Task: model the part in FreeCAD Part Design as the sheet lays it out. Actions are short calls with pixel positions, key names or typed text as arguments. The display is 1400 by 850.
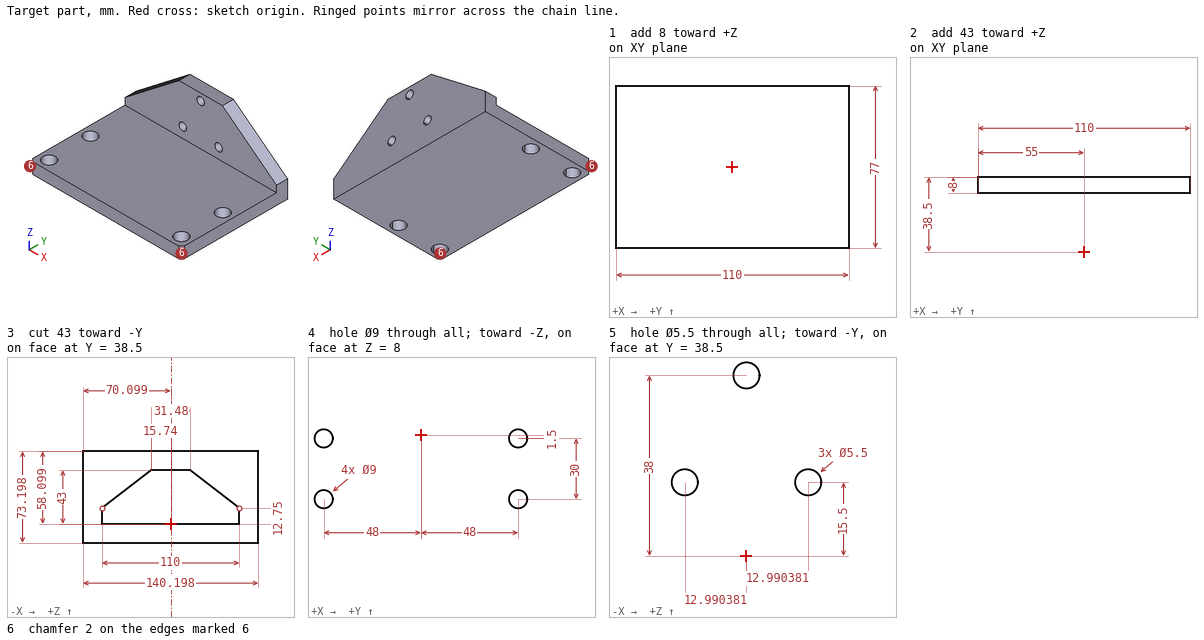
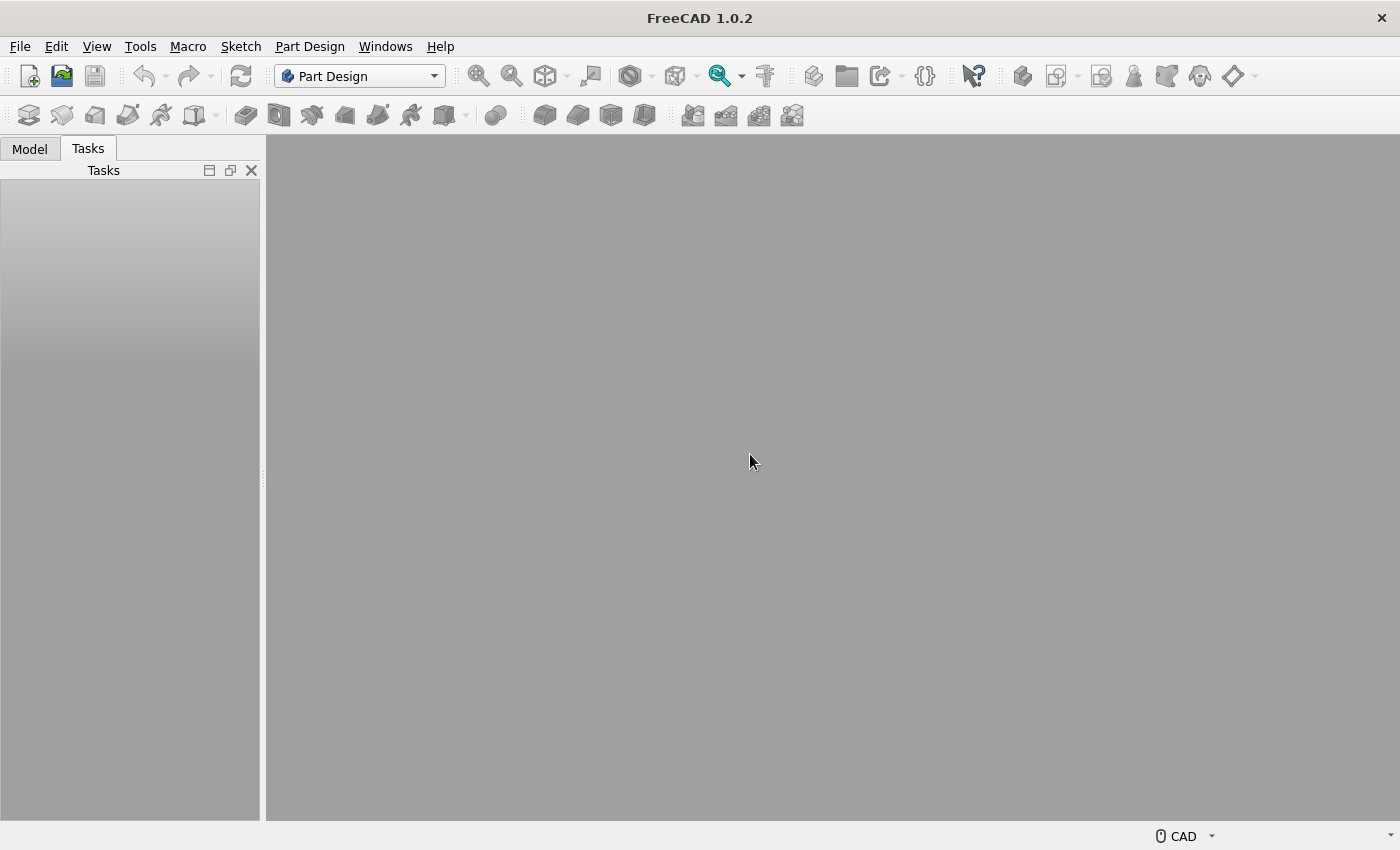
key(ctrl+n)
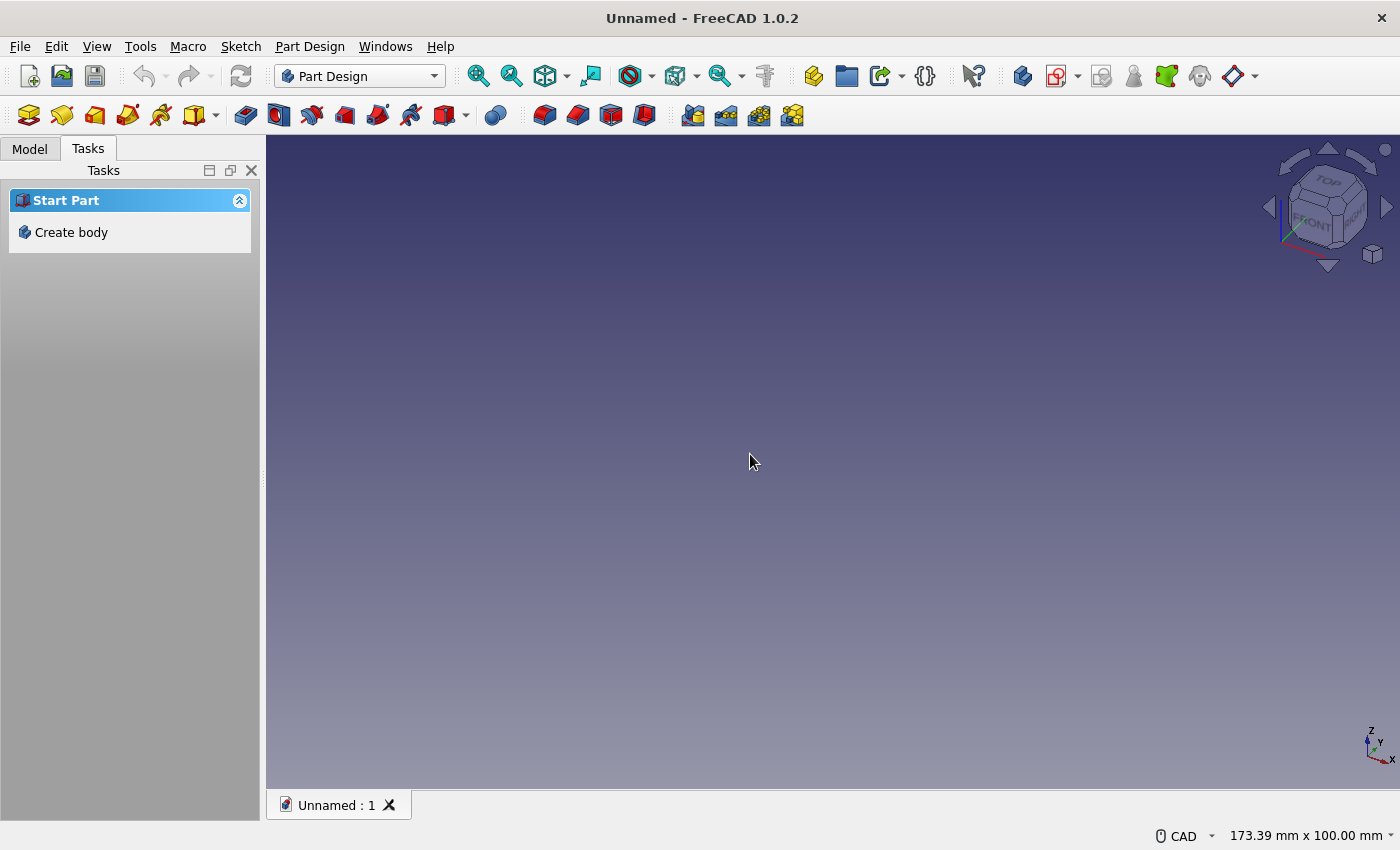
click(1056, 76)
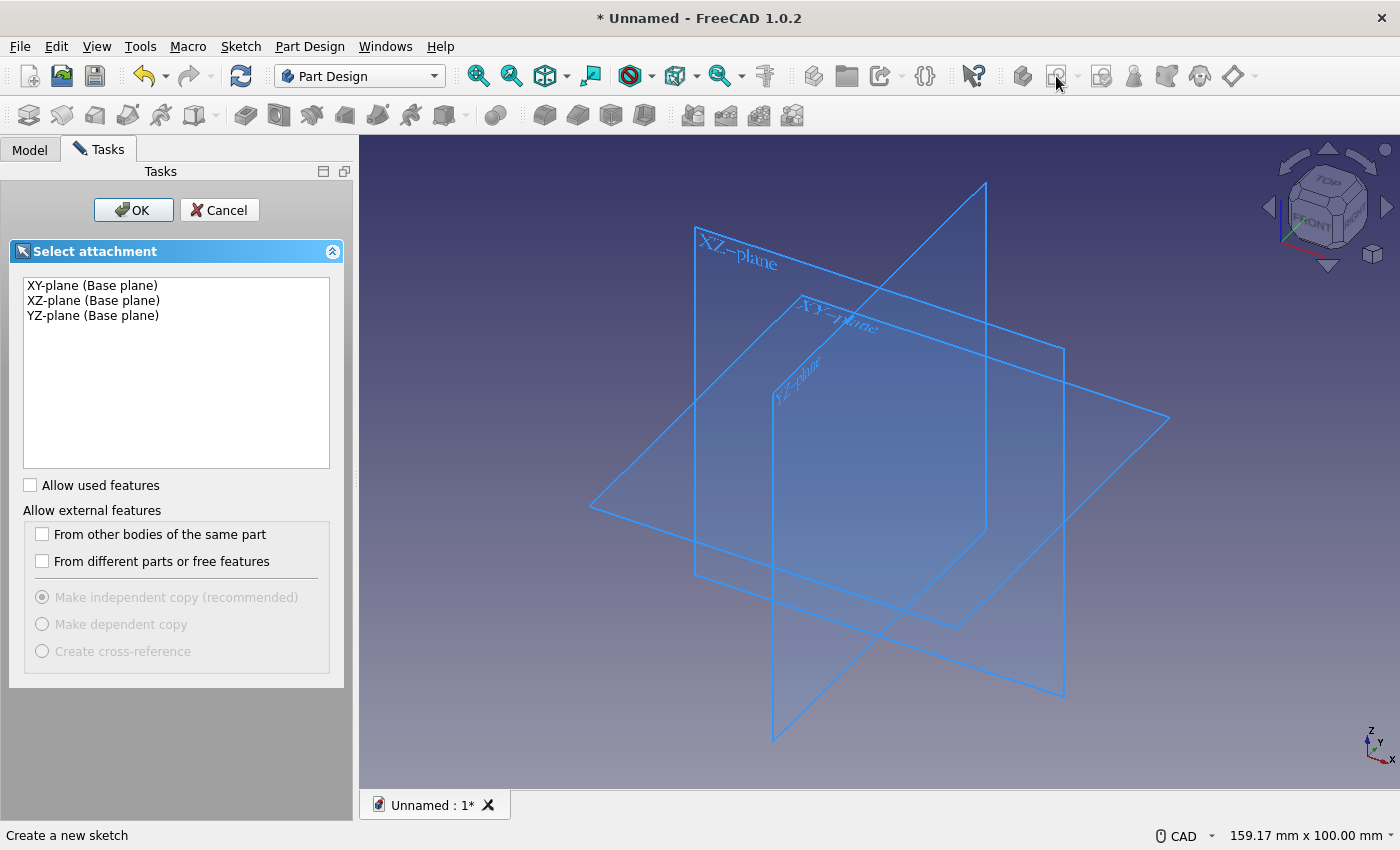
click(84, 286)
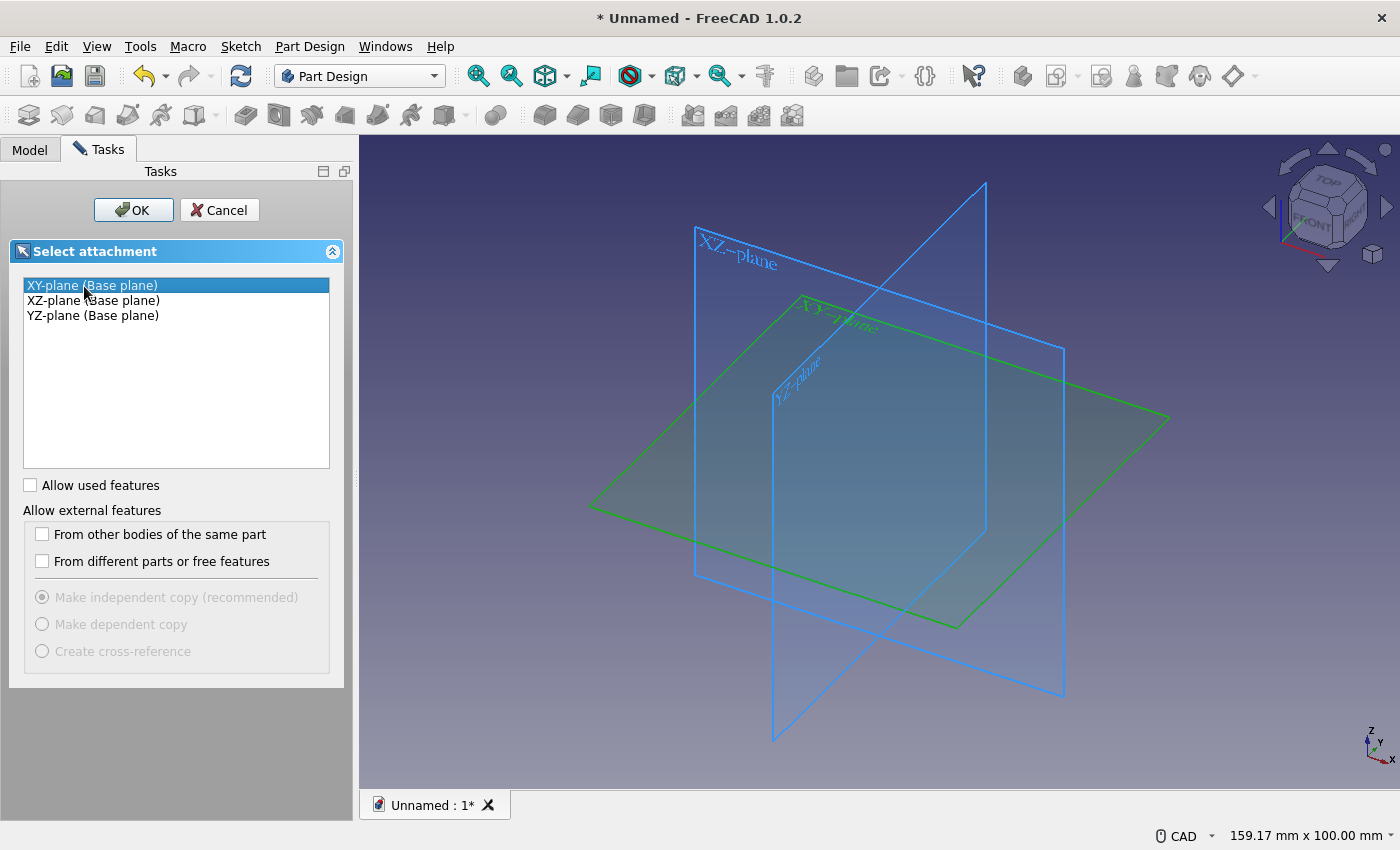
click(134, 210)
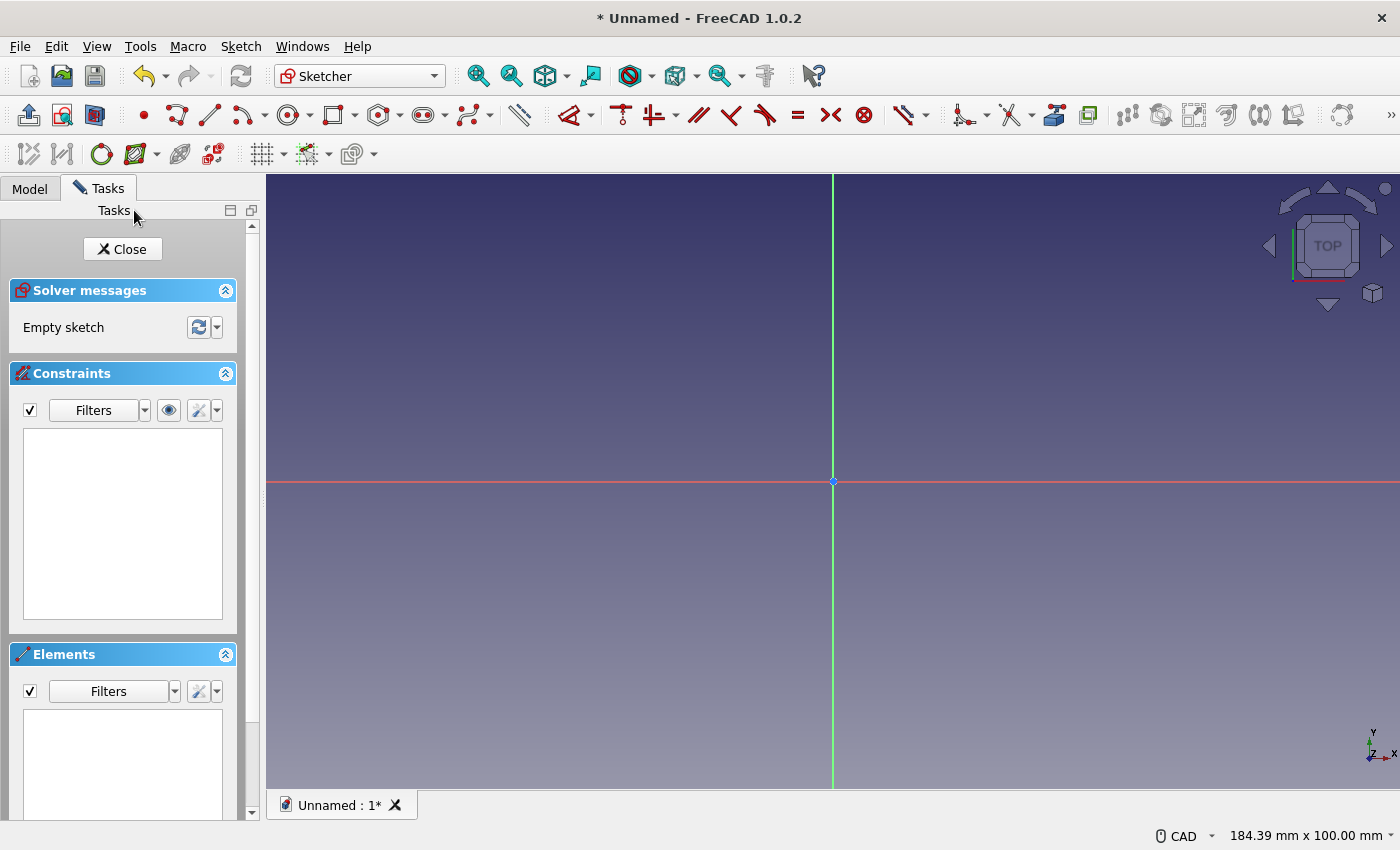
key(g)
key(v)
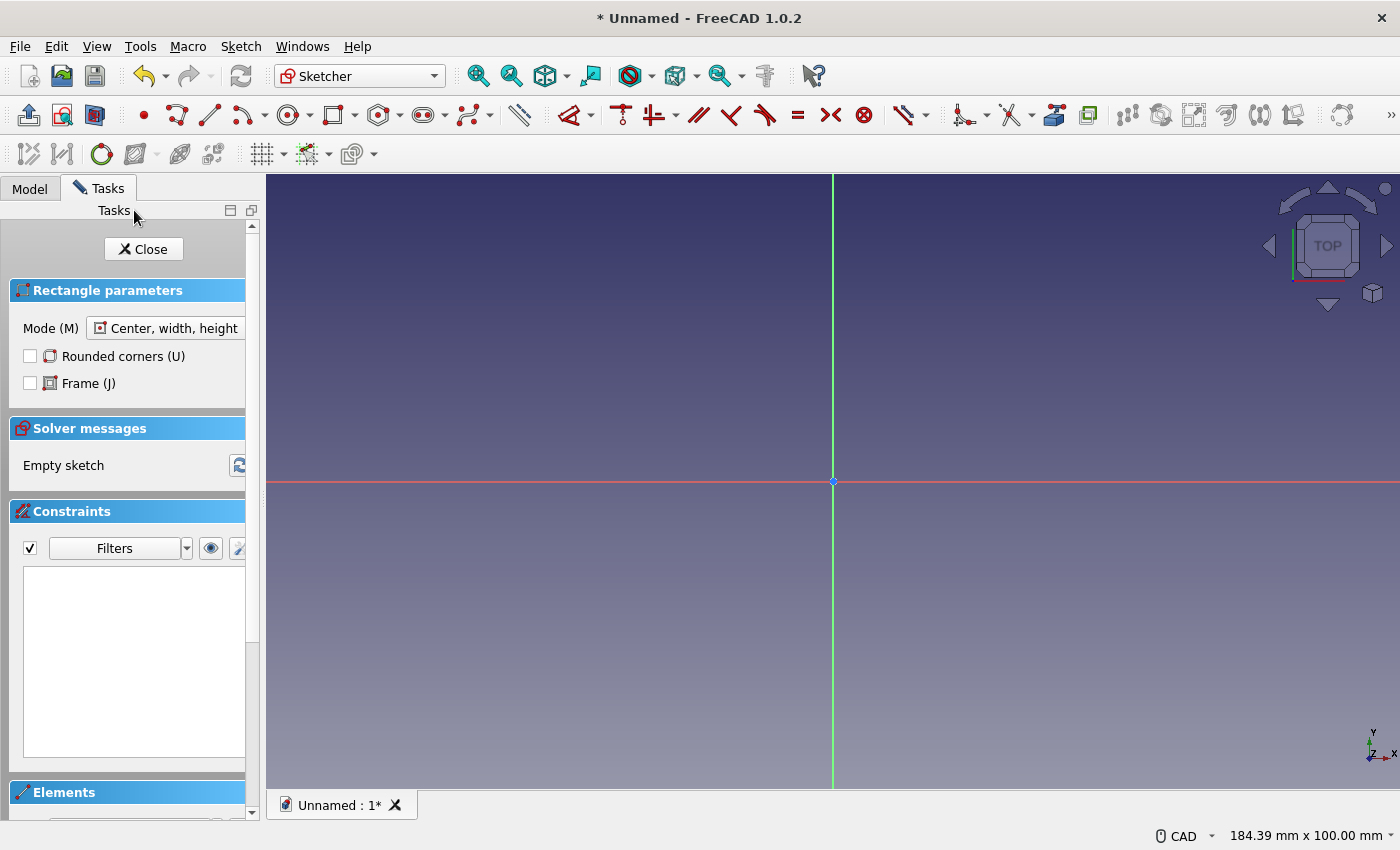
click(833, 482)
click(1171, 245)
key(Escape)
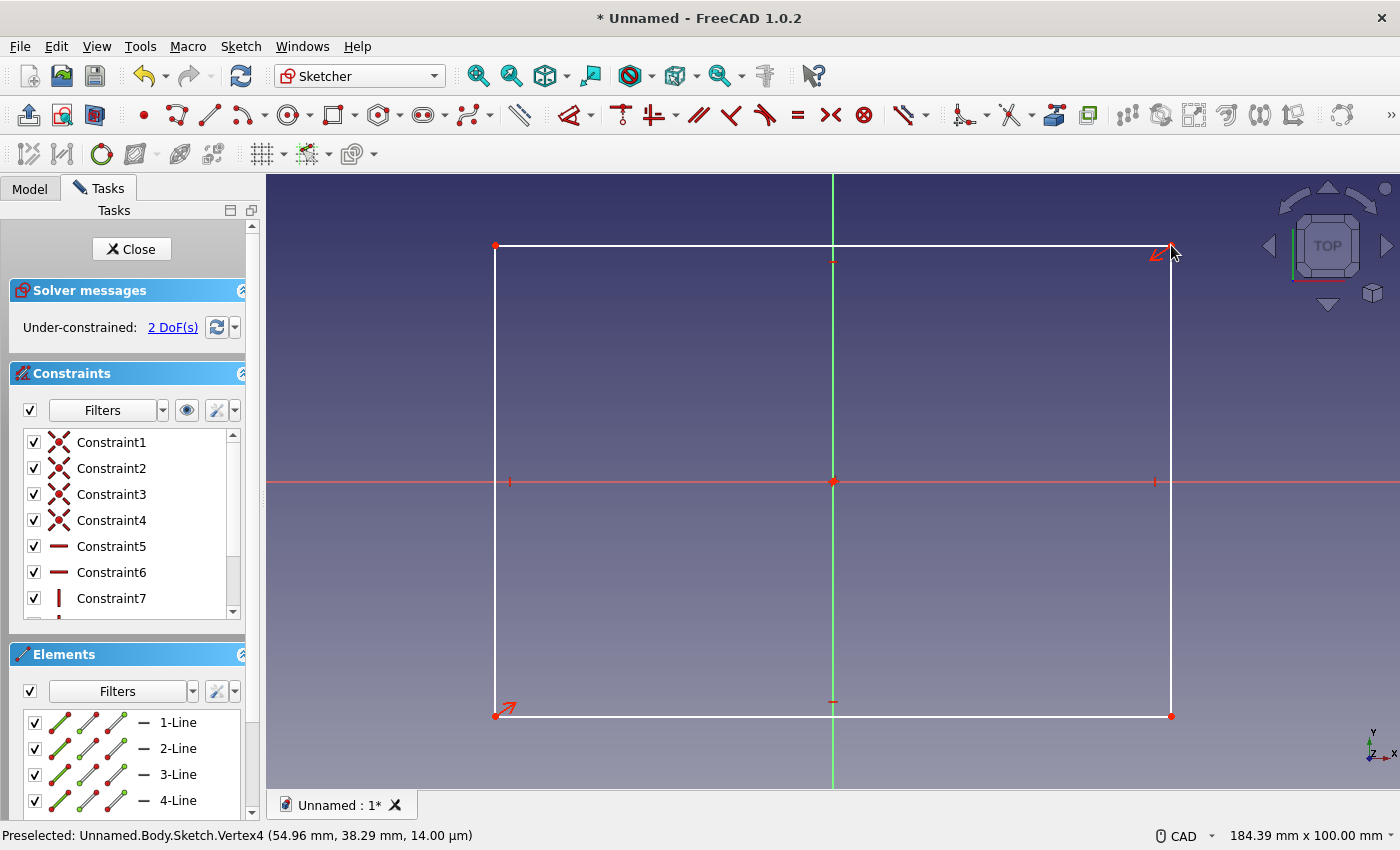
click(1171, 576)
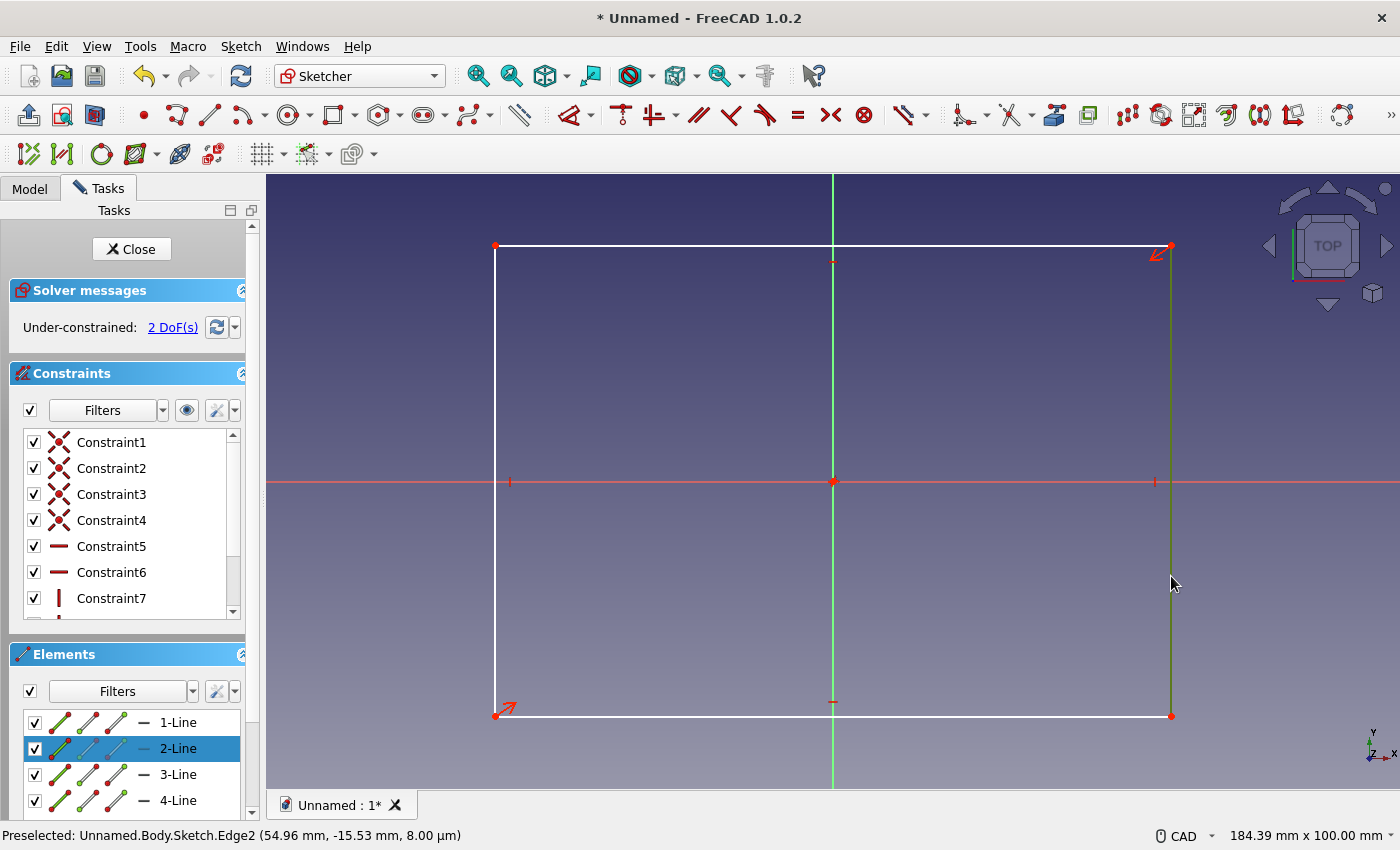
click(590, 116)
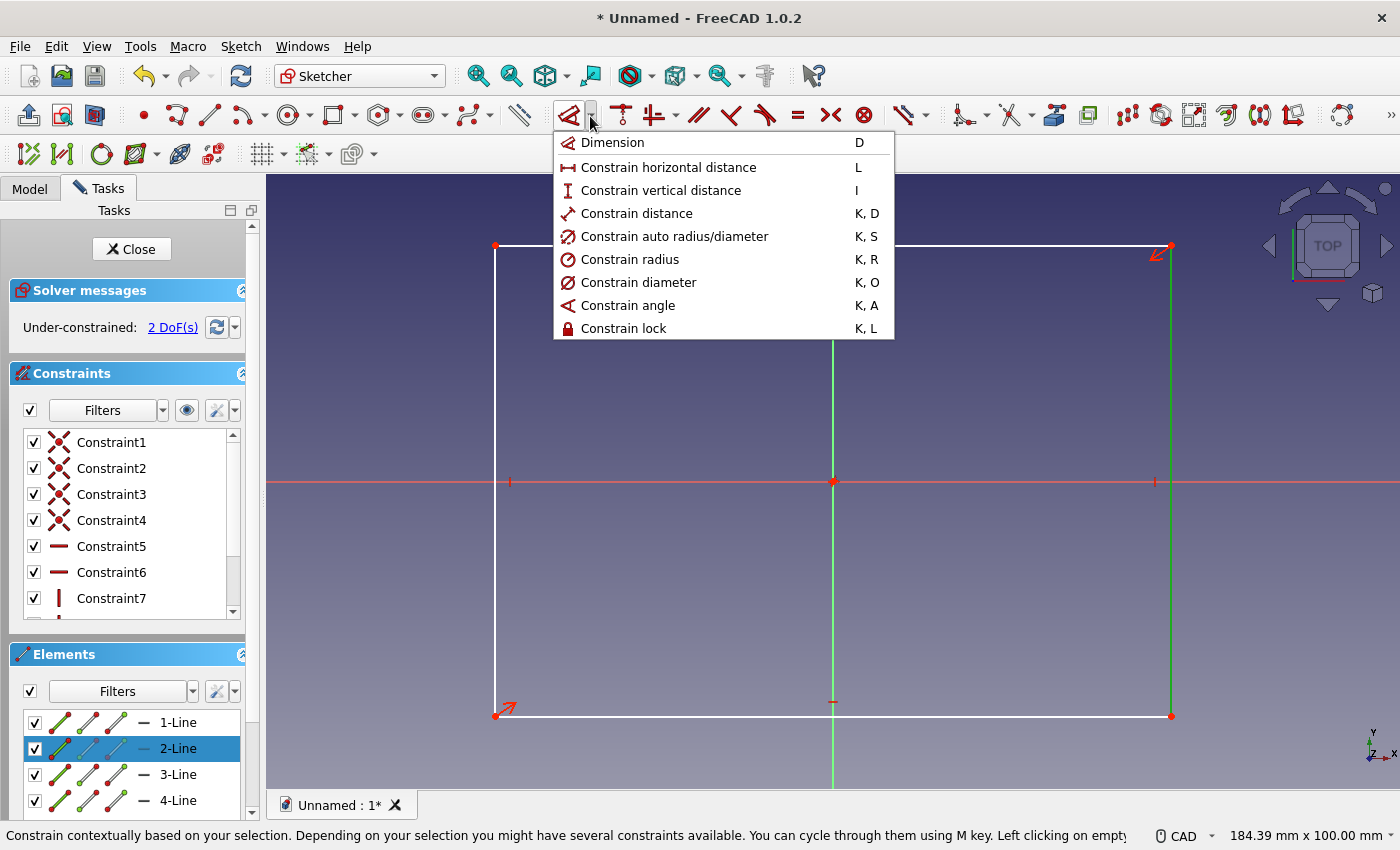
click(724, 190)